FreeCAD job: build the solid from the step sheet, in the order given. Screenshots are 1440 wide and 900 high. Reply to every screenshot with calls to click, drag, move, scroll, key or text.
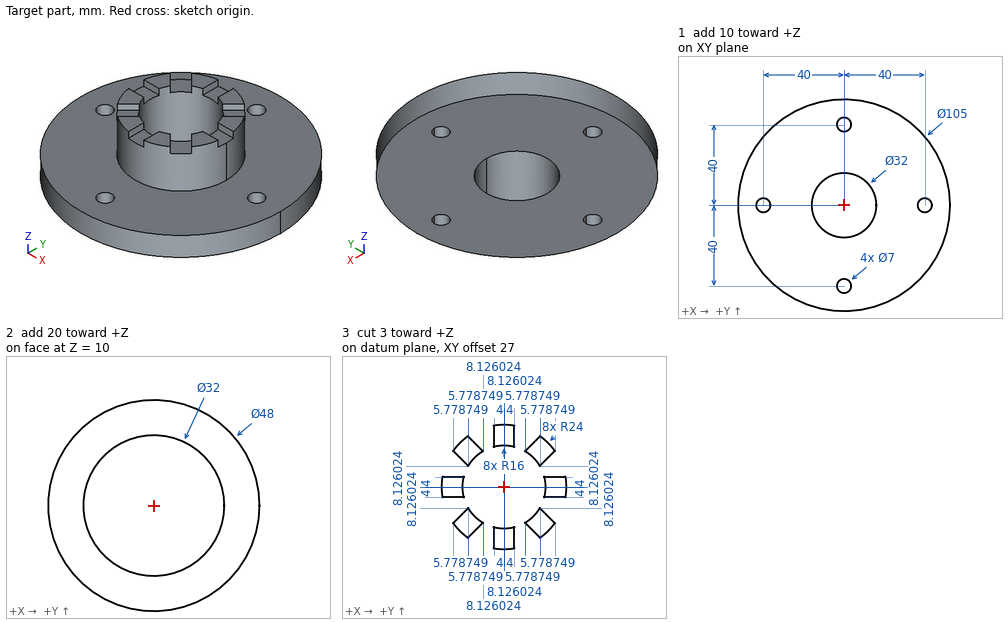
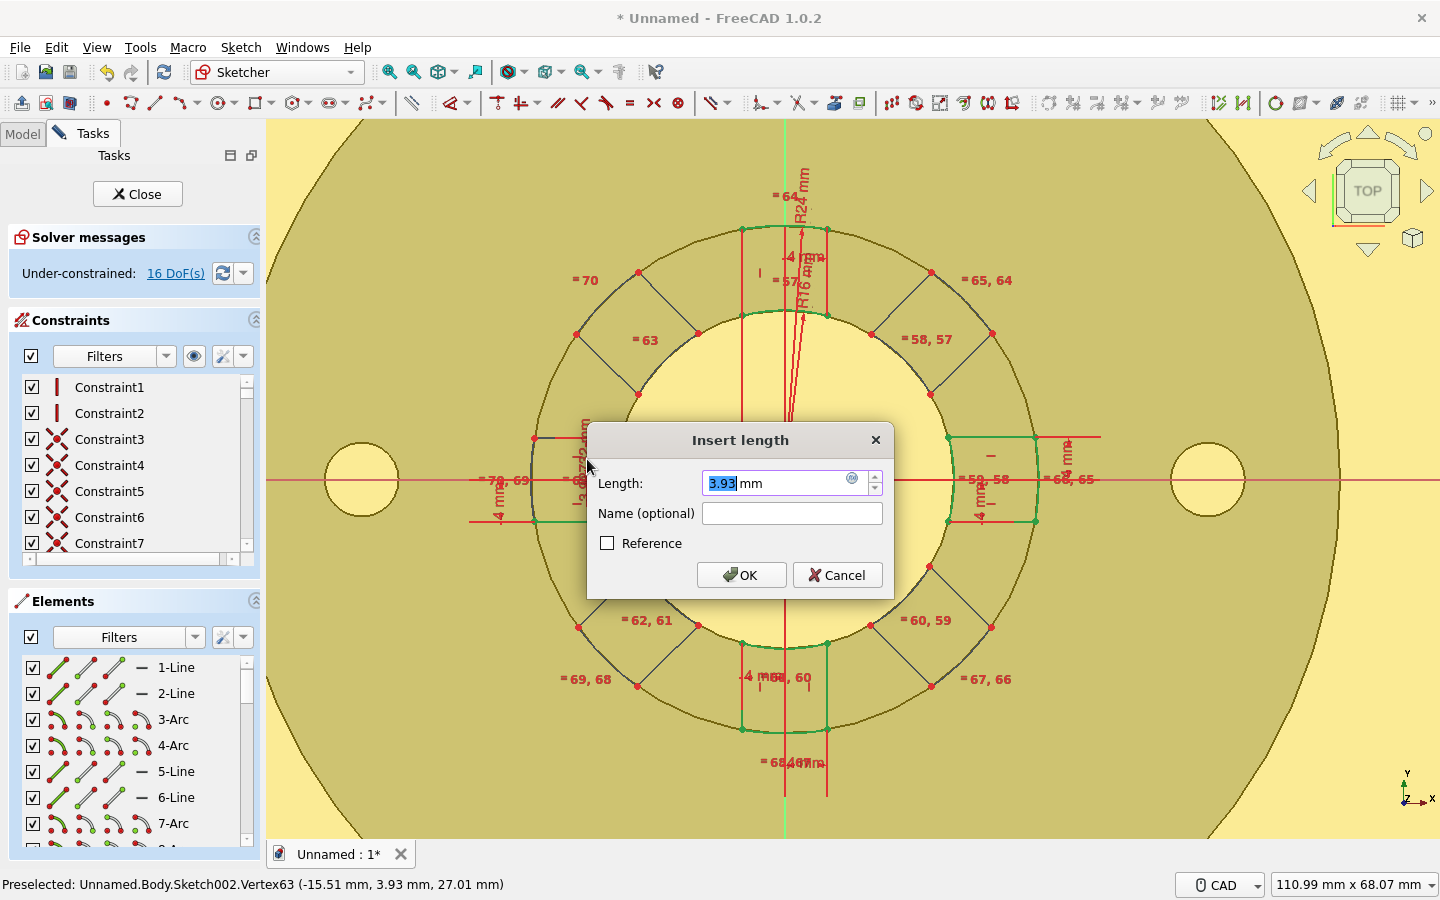
text(4)
key(Return)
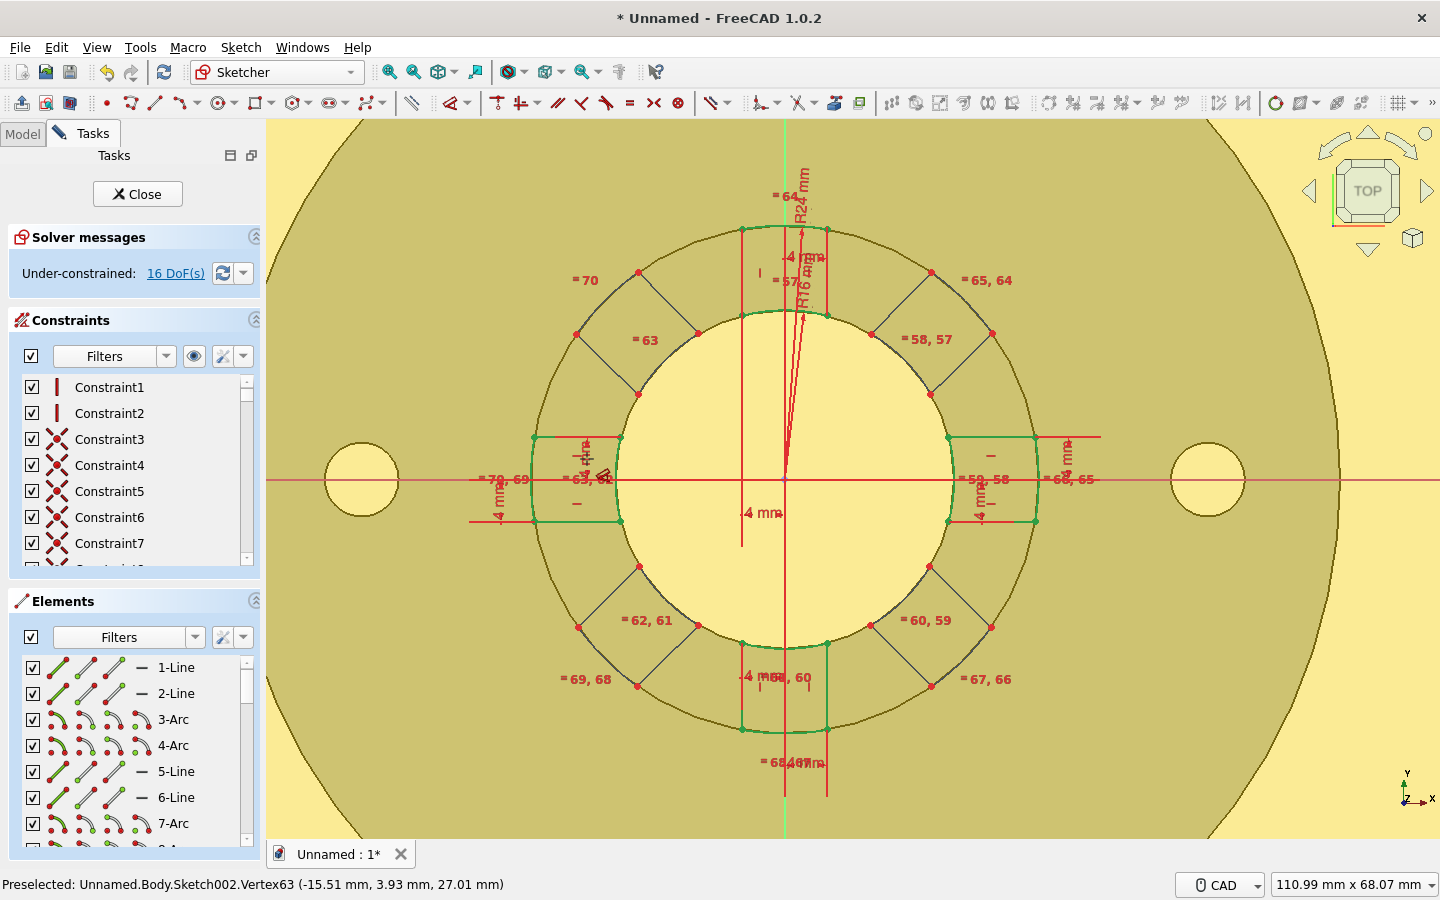
click(871, 334)
click(848, 514)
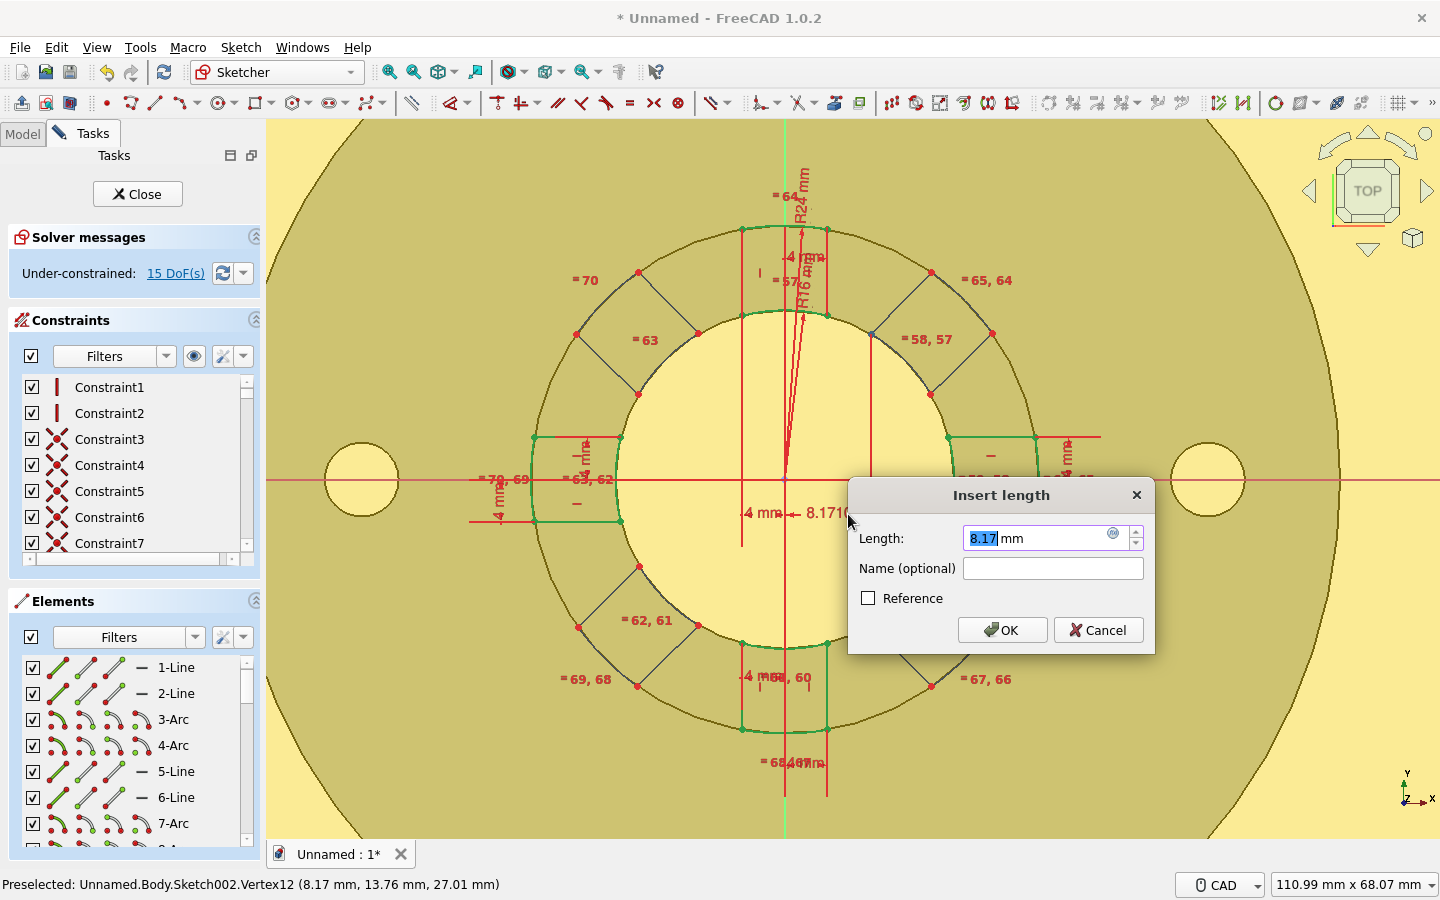
text(8.126024)
key(Return)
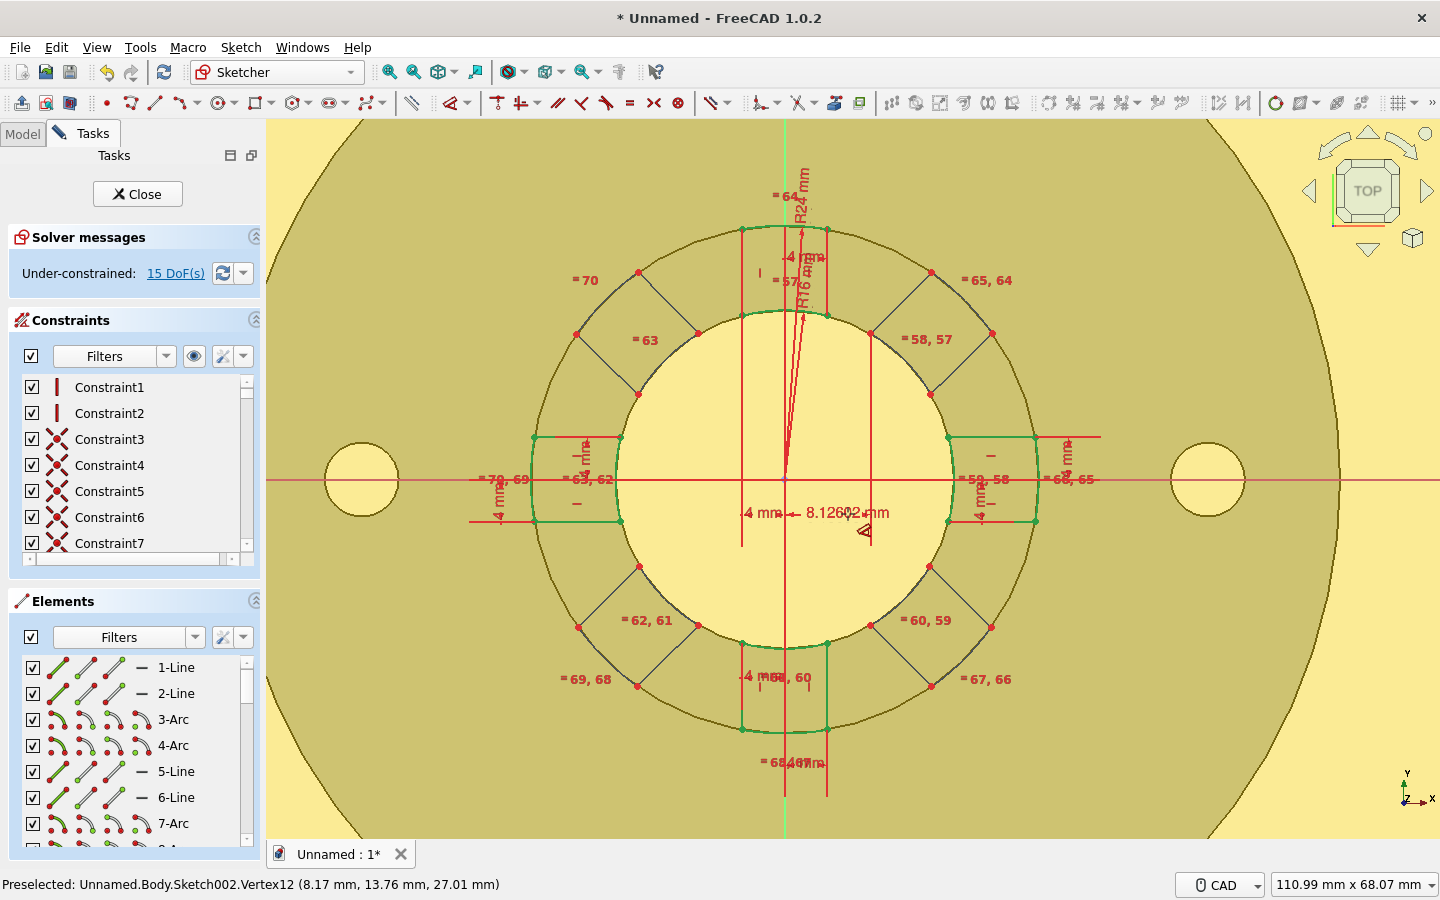
click(931, 394)
click(965, 417)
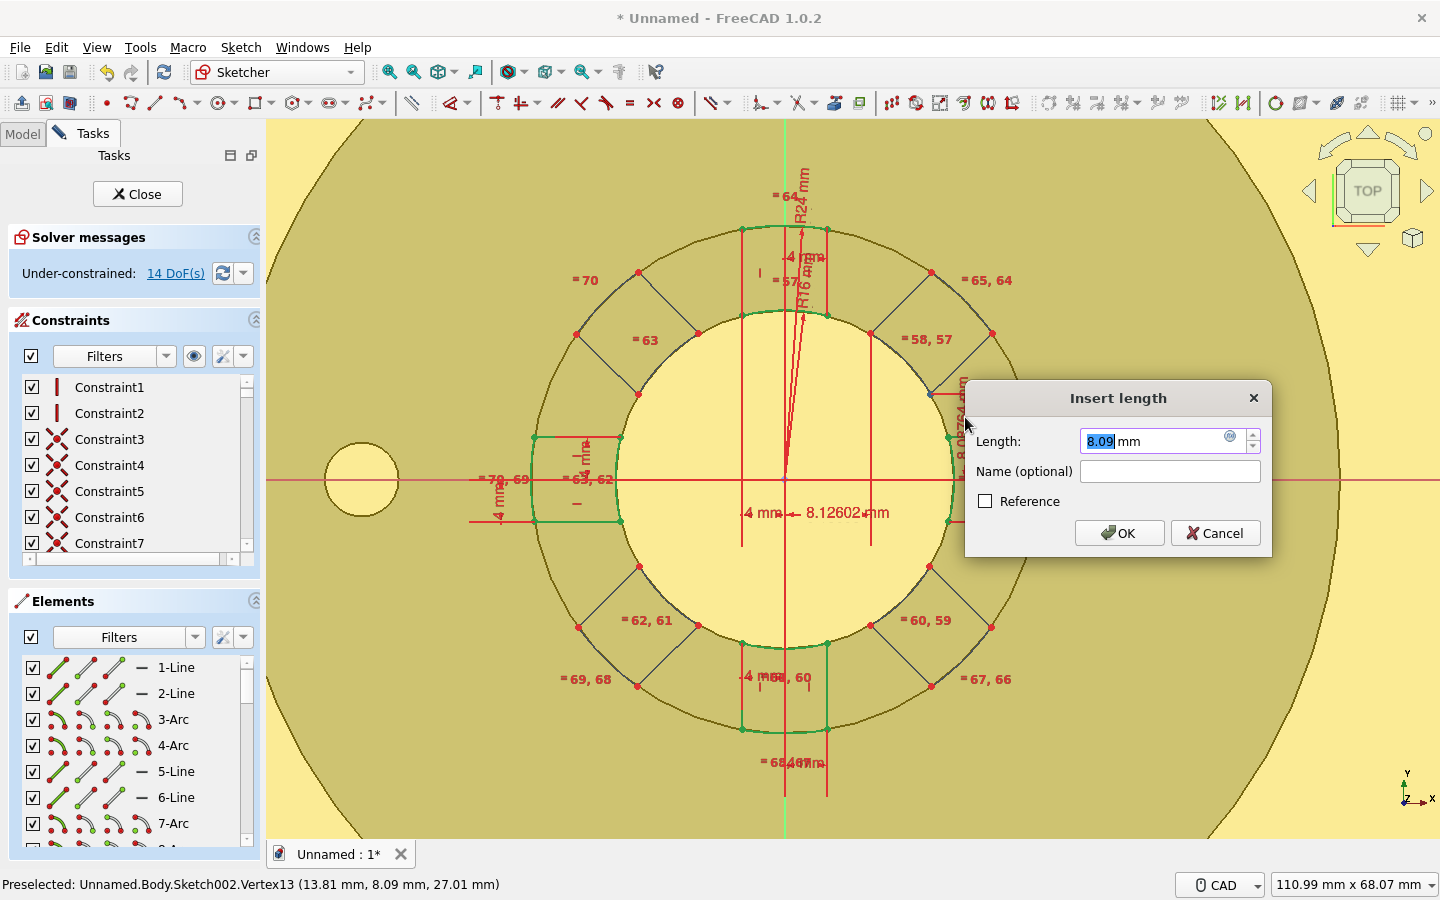
text(8.126024)
key(Return)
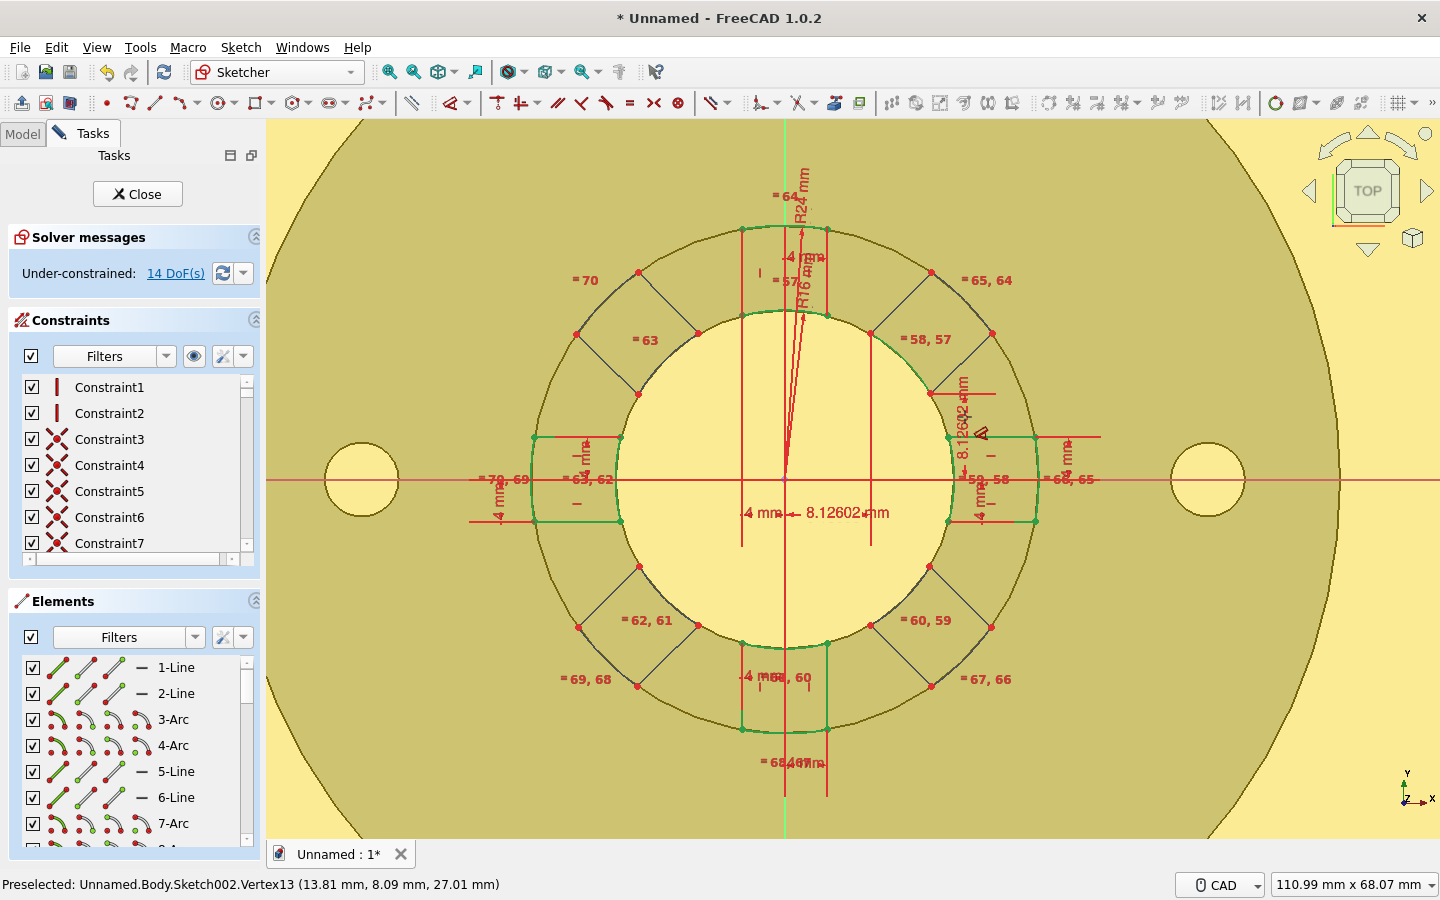
click(930, 567)
click(964, 543)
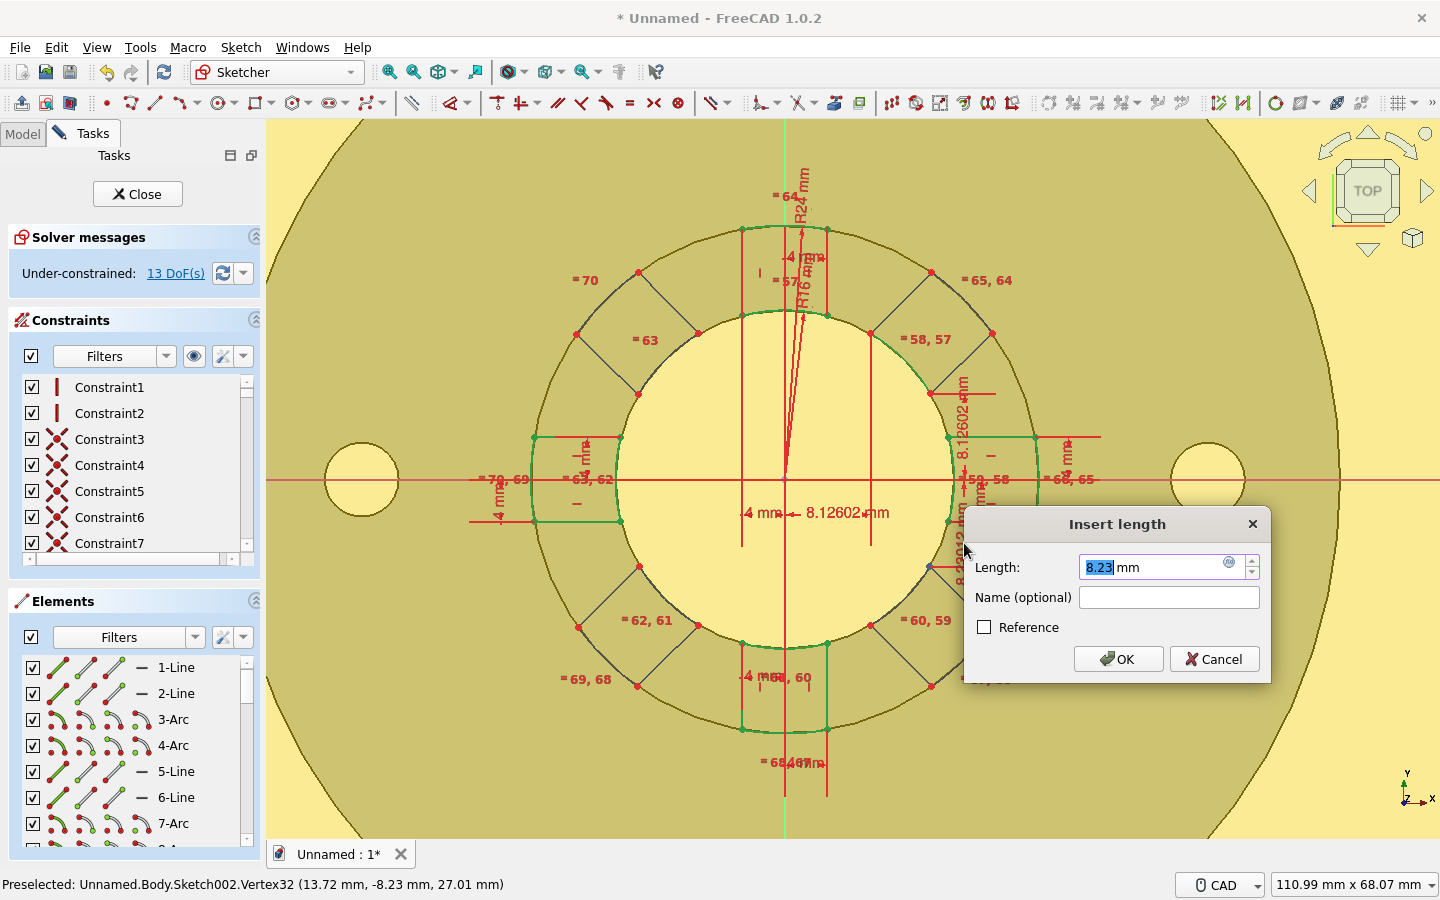
text(8.126024)
key(Return)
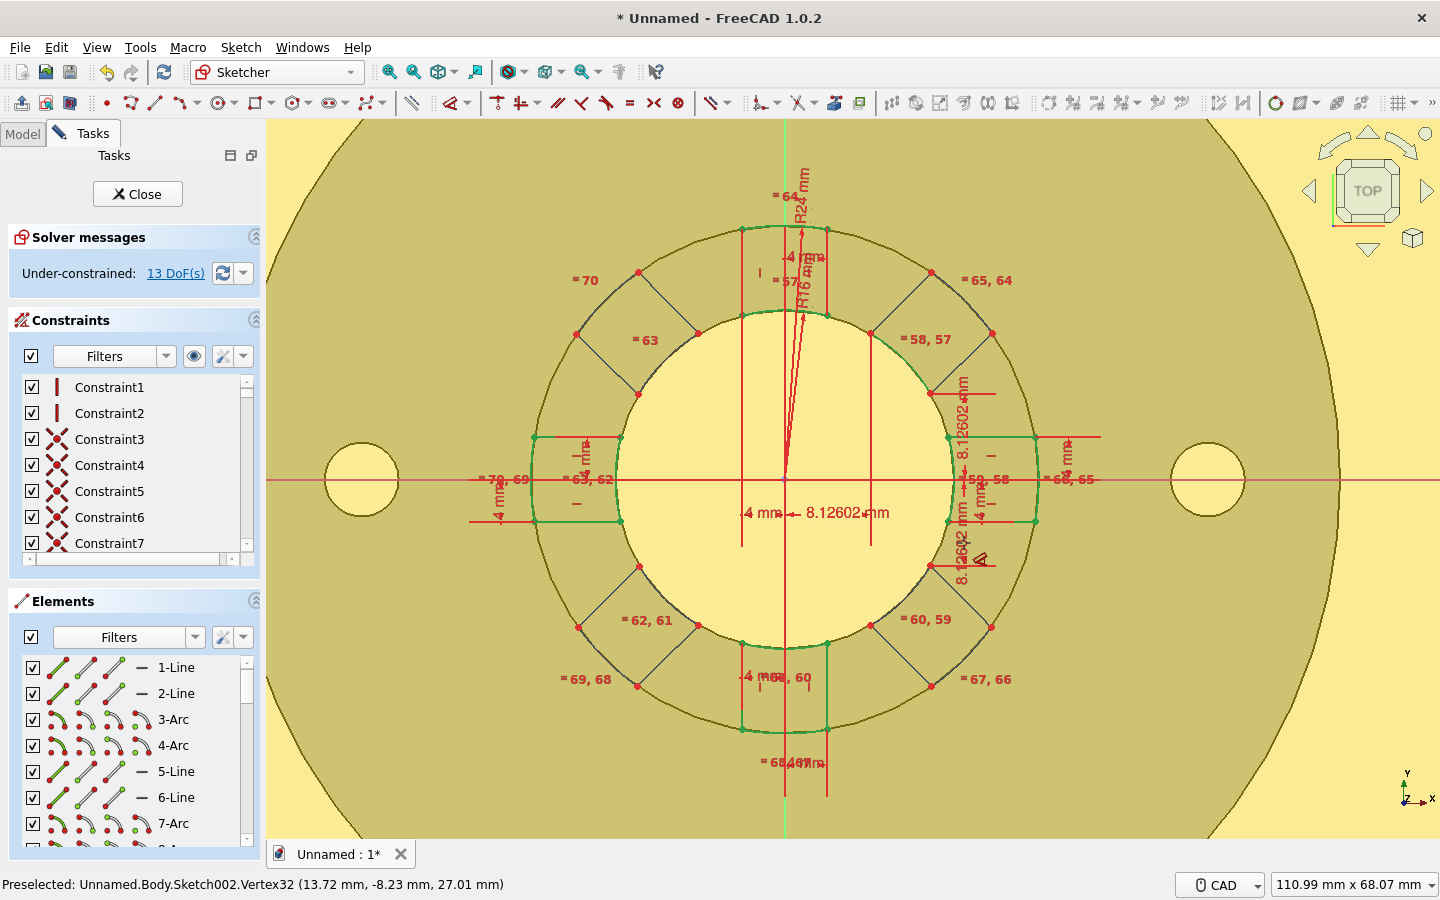
click(871, 625)
click(848, 659)